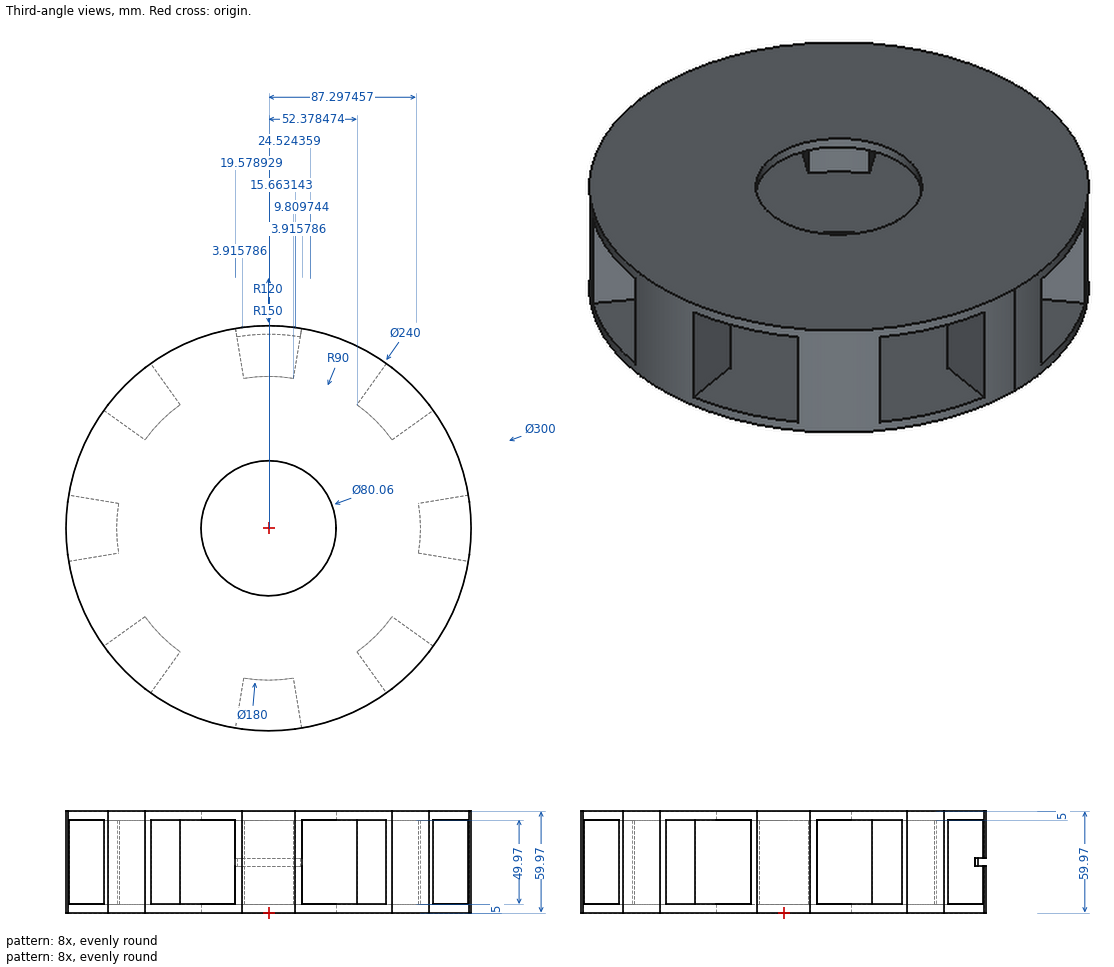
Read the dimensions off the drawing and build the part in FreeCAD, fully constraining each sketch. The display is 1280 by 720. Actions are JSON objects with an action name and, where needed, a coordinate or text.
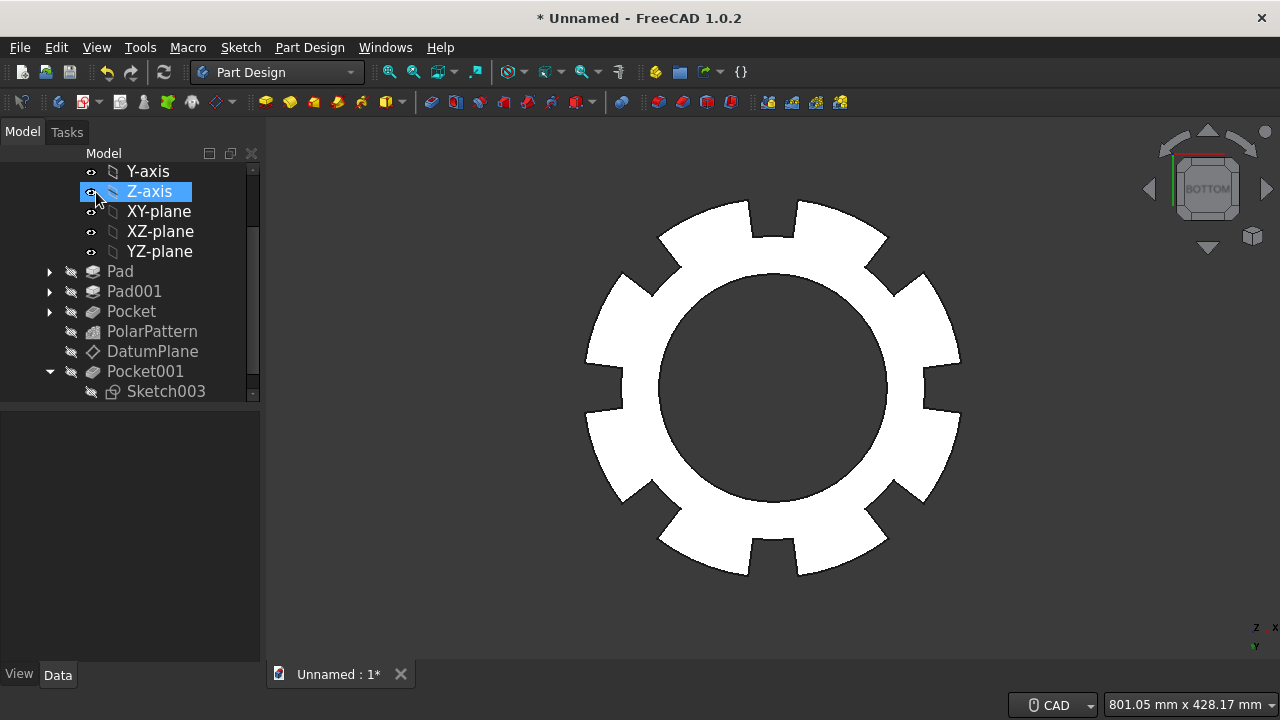
{"action": "scroll", "coordinate": [160, 287], "scroll_direction": "down", "scroll_amount": 3}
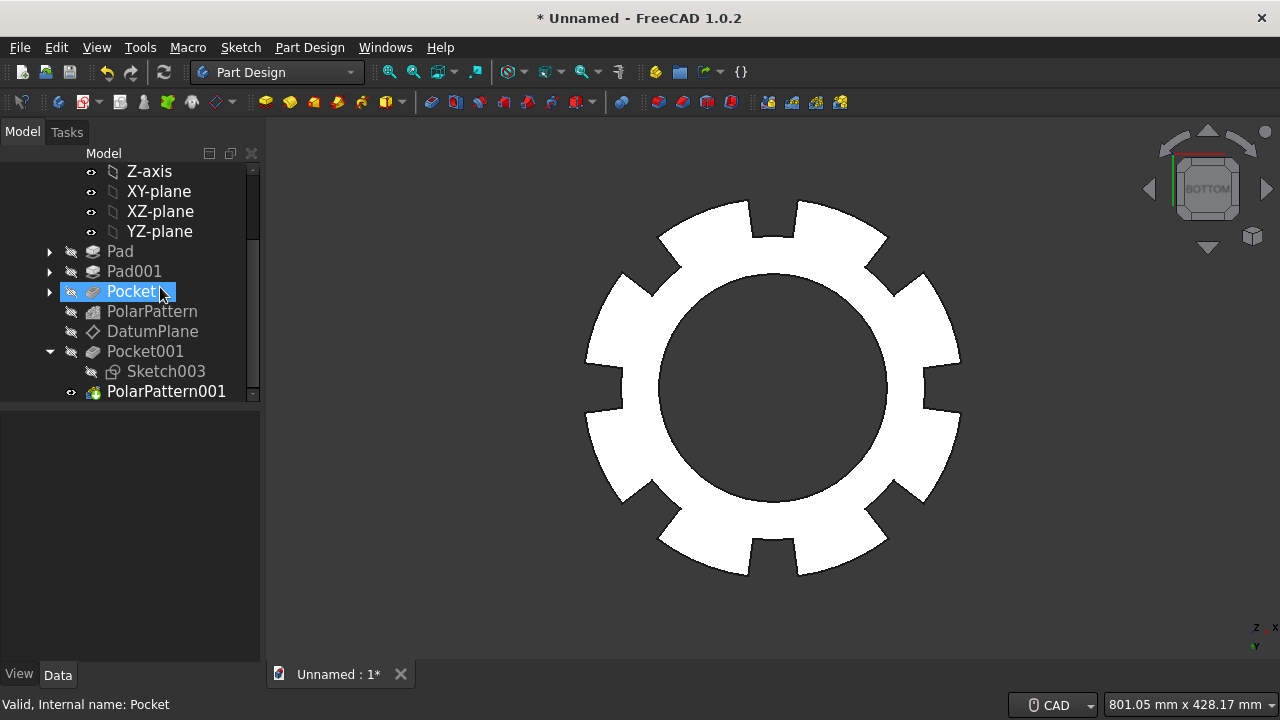
{"action": "scroll", "coordinate": [160, 287], "scroll_direction": "up", "scroll_amount": 15}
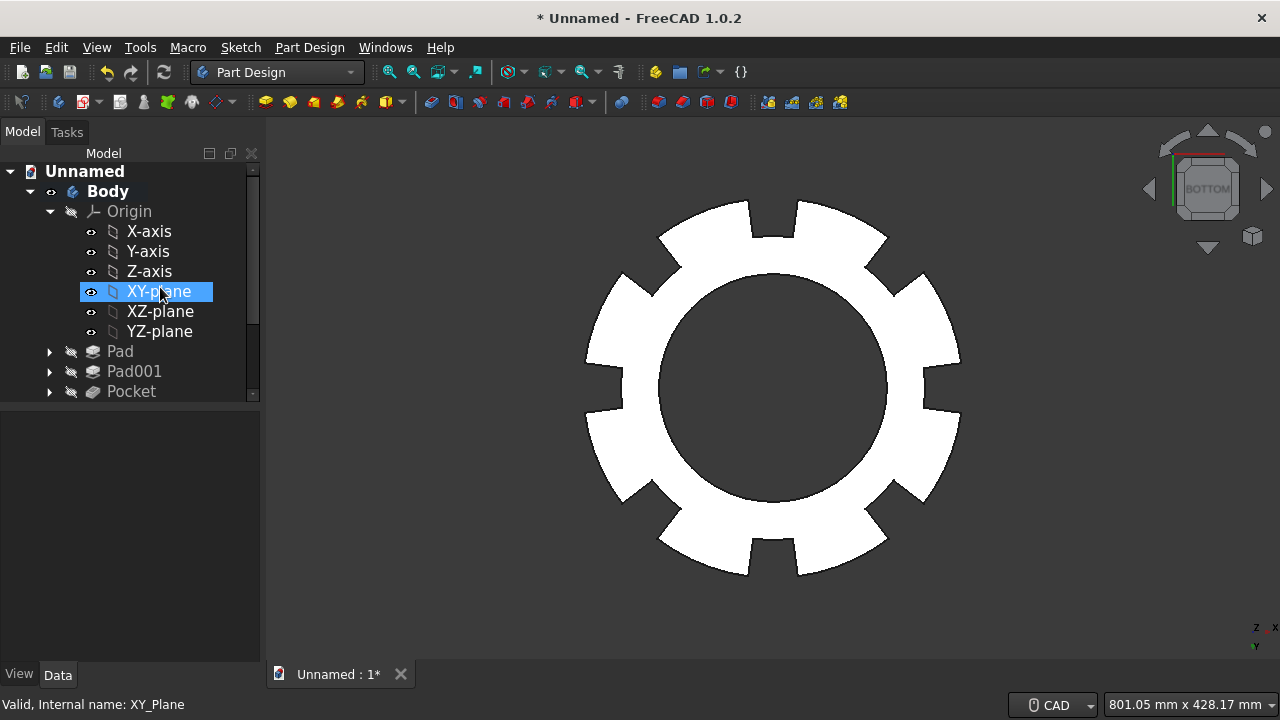
{"action": "left_click", "coordinate": [136, 292]}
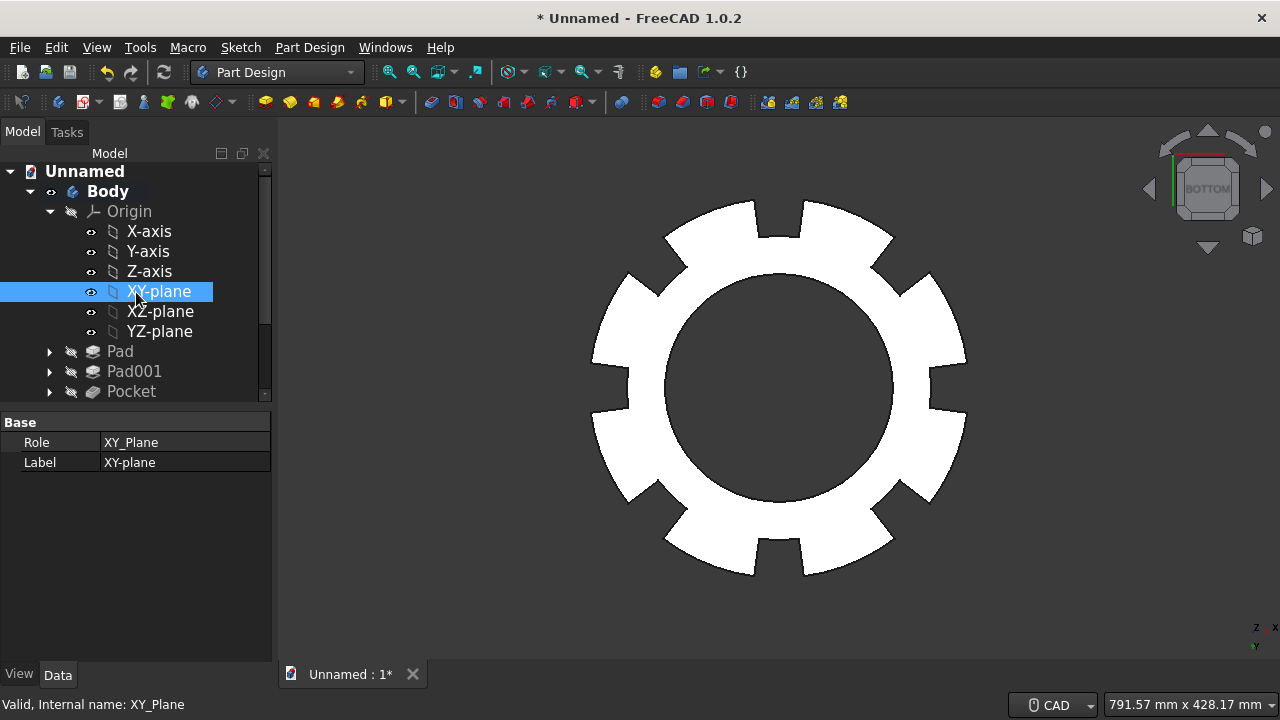
{"action": "left_click", "coordinate": [216, 102]}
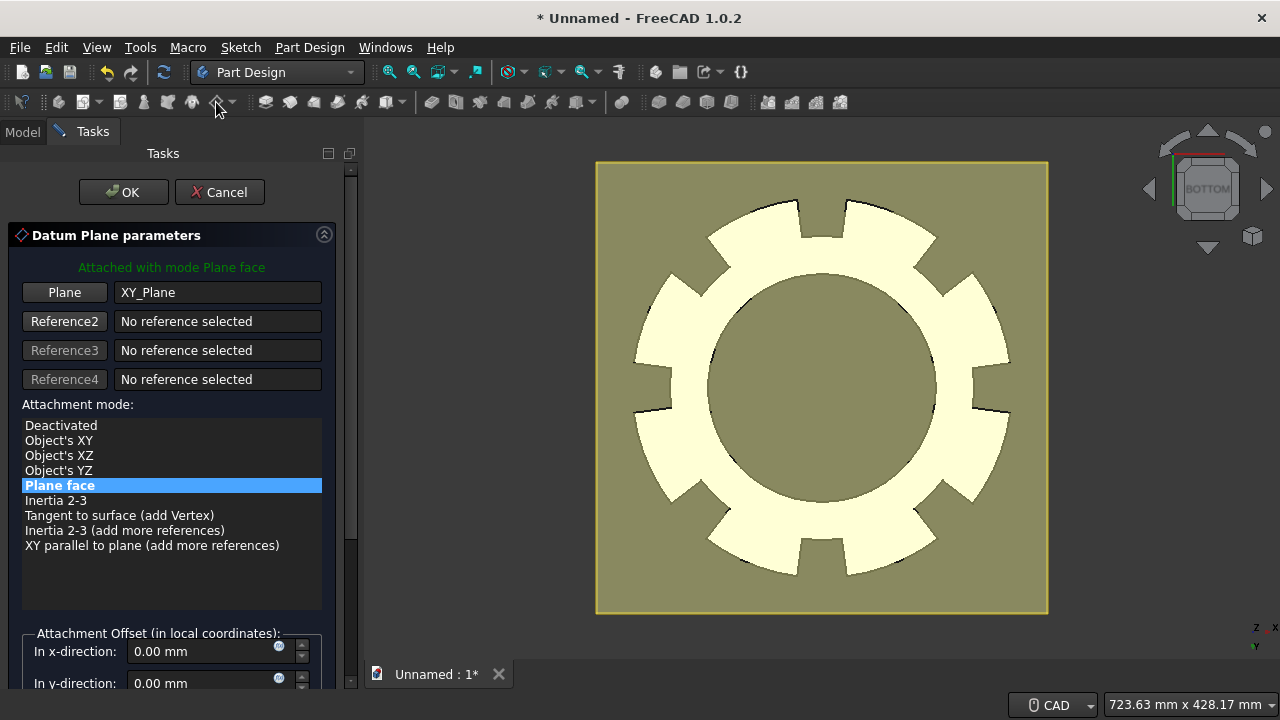
{"action": "scroll", "coordinate": [351, 426], "scroll_direction": "down", "scroll_amount": 2}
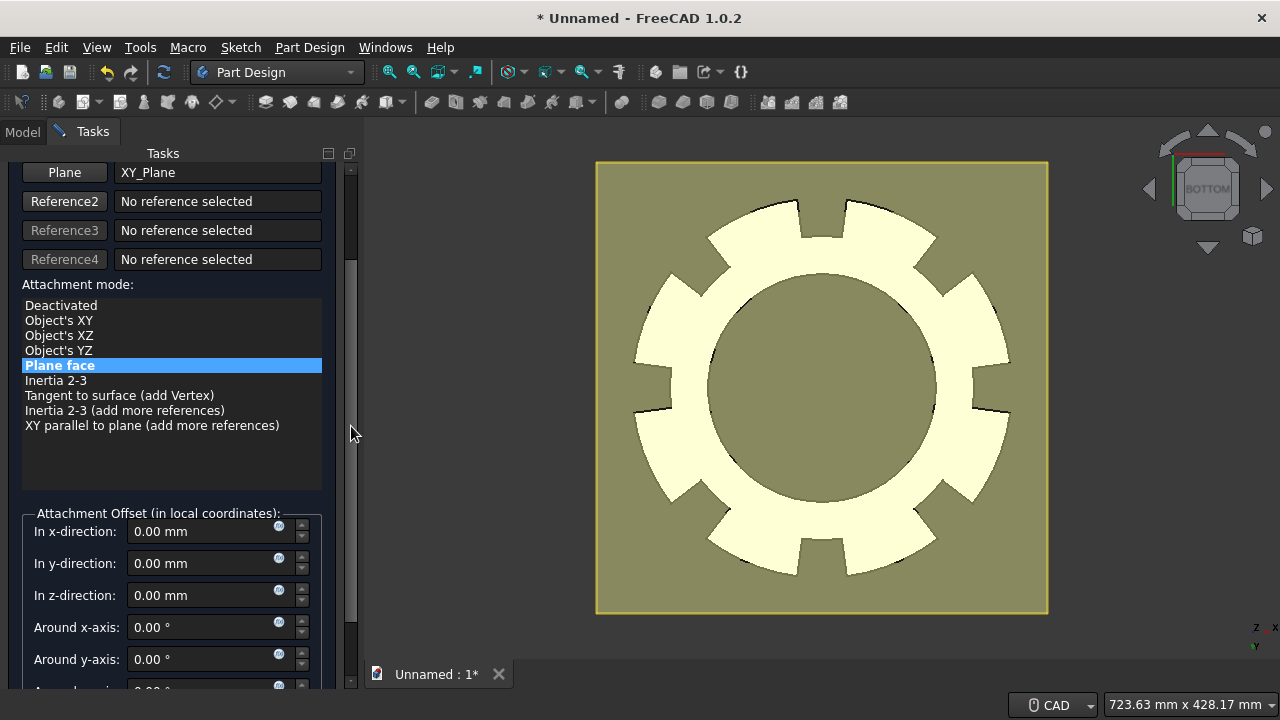
{"action": "triple_click", "coordinate": [210, 595]}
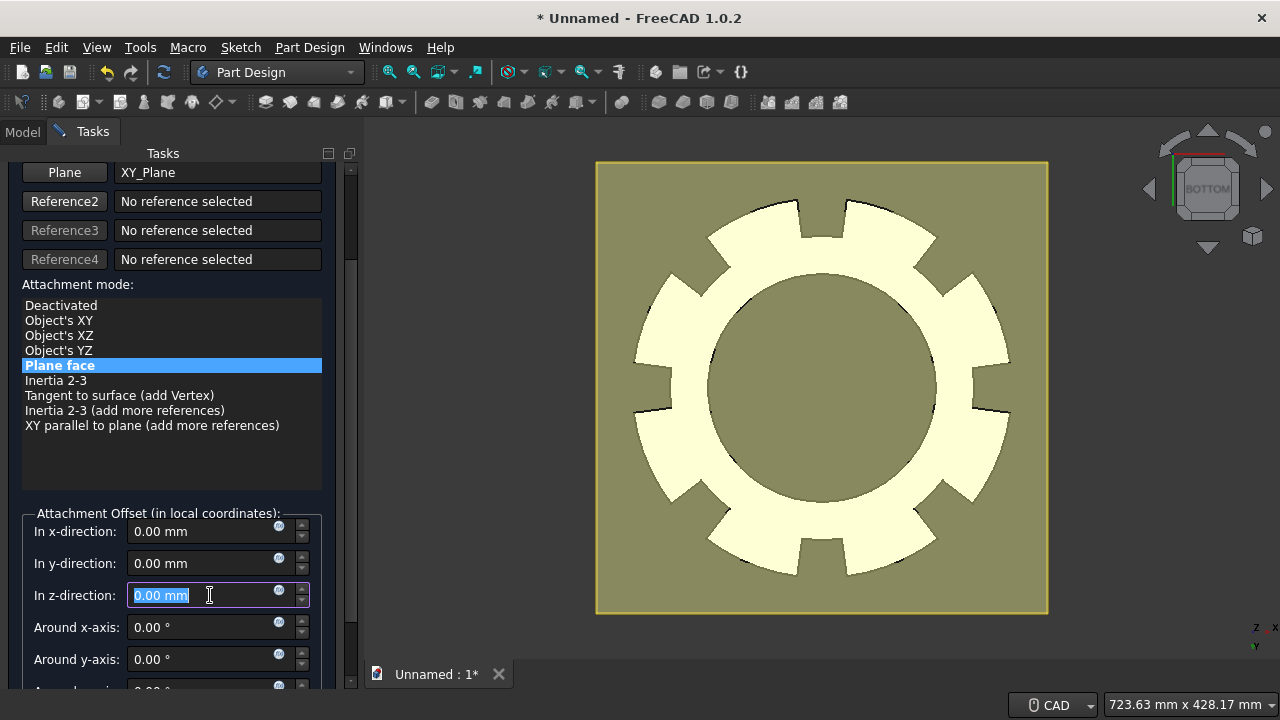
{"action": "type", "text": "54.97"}
{"action": "key", "text": "Tab"}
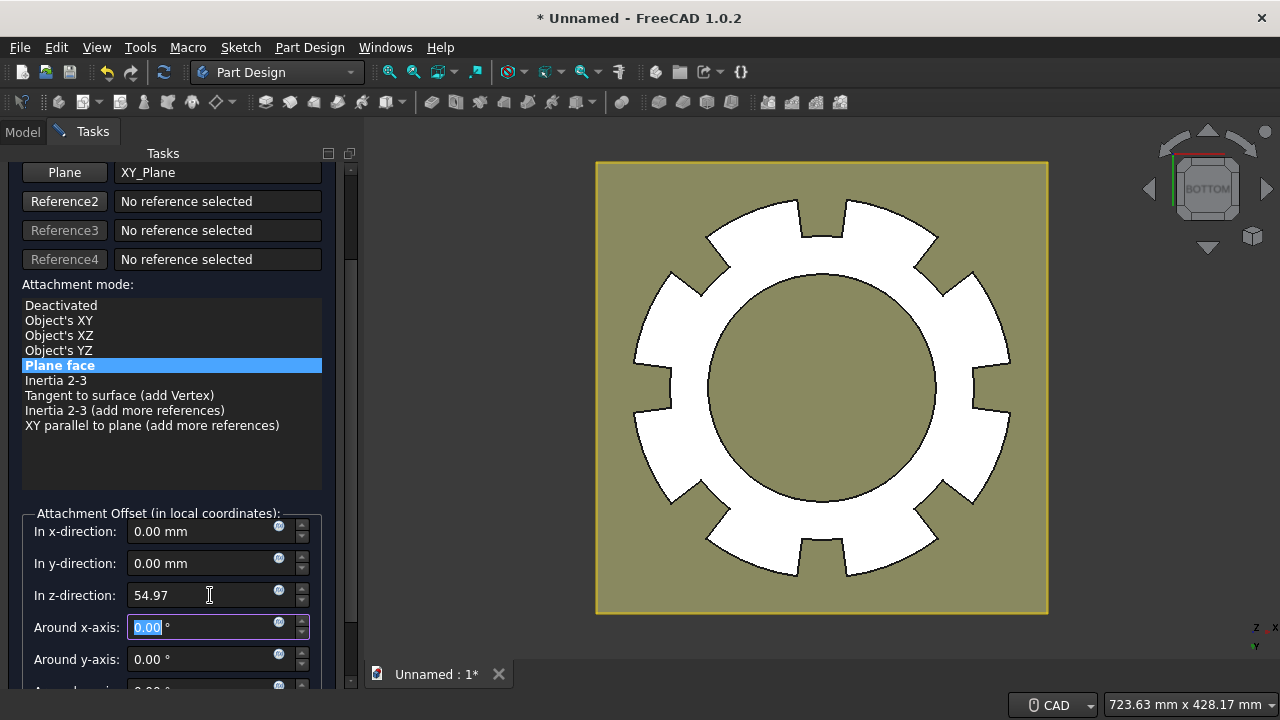
{"action": "scroll", "coordinate": [351, 426], "scroll_direction": "up", "scroll_amount": 3}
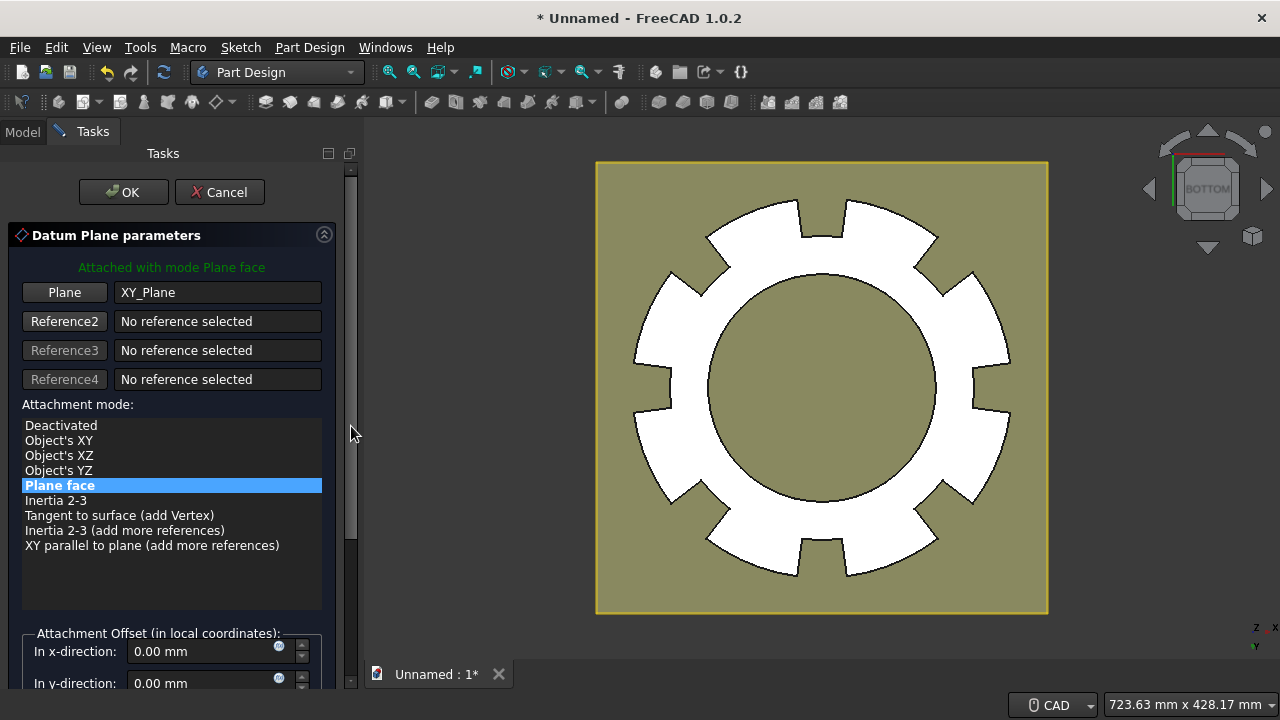
{"action": "left_click", "coordinate": [124, 192]}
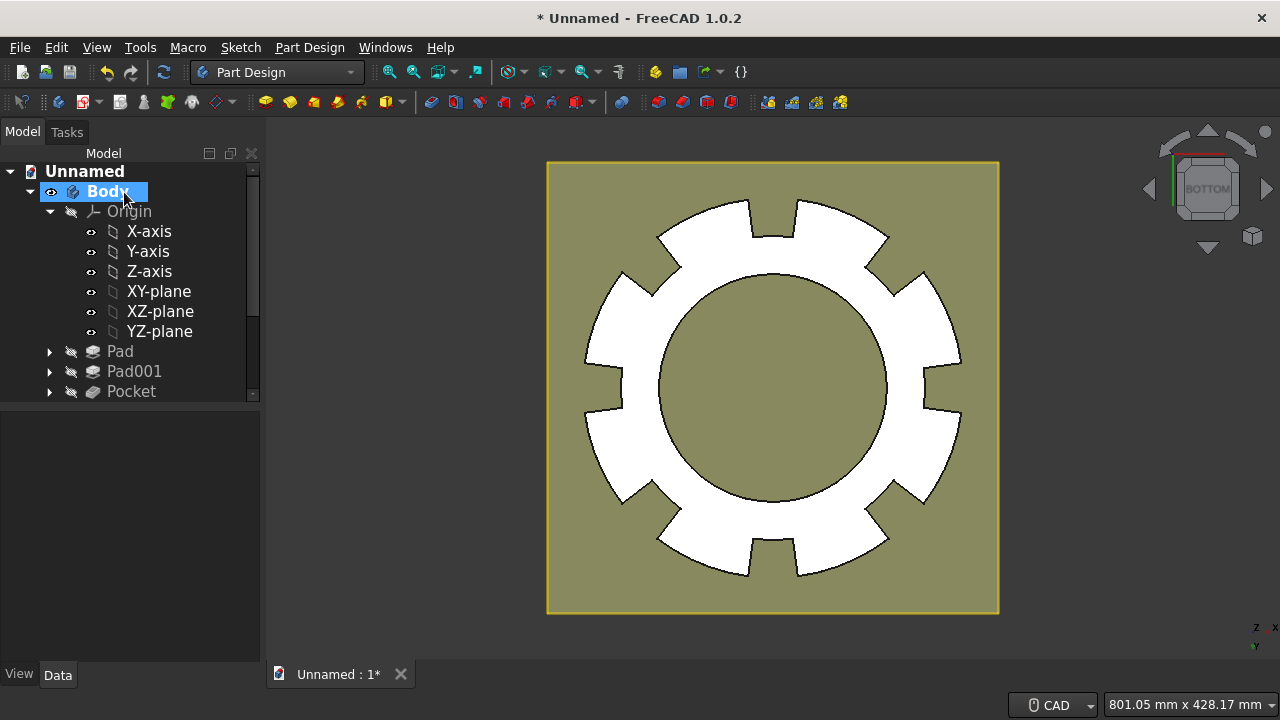
{"action": "scroll", "coordinate": [100, 287], "scroll_direction": "down", "scroll_amount": 3}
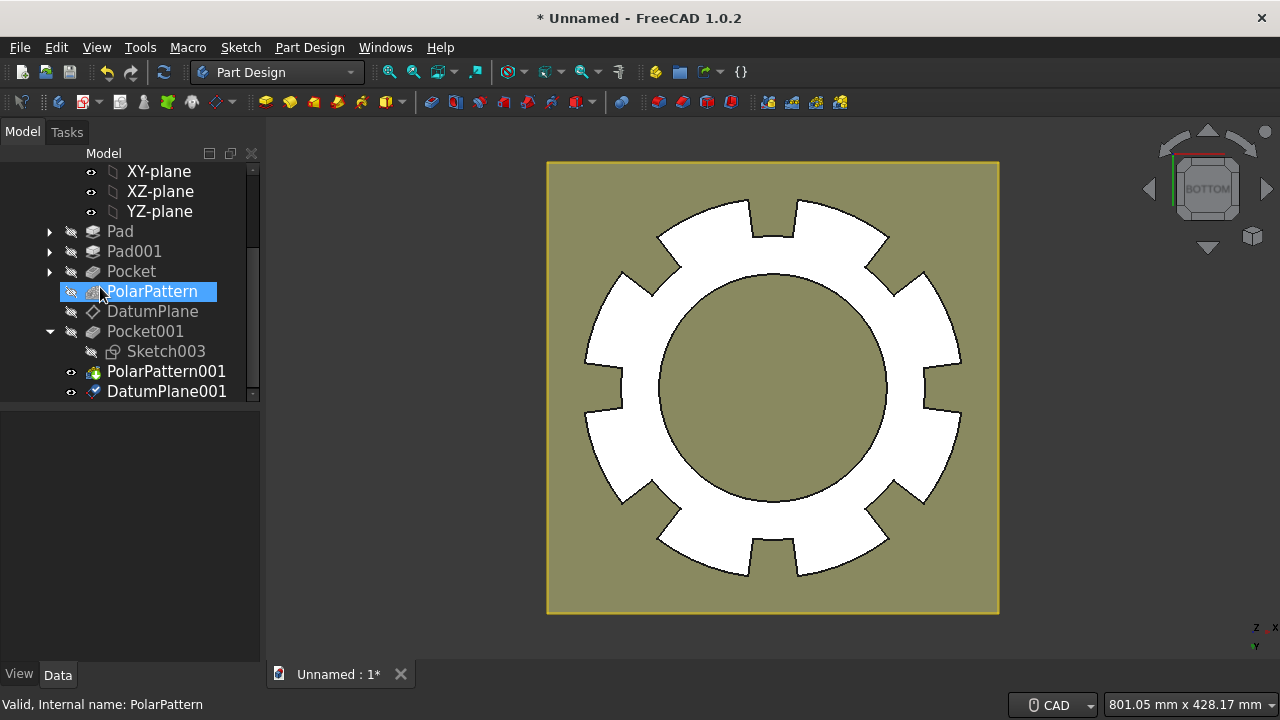
{"action": "left_click", "coordinate": [116, 392]}